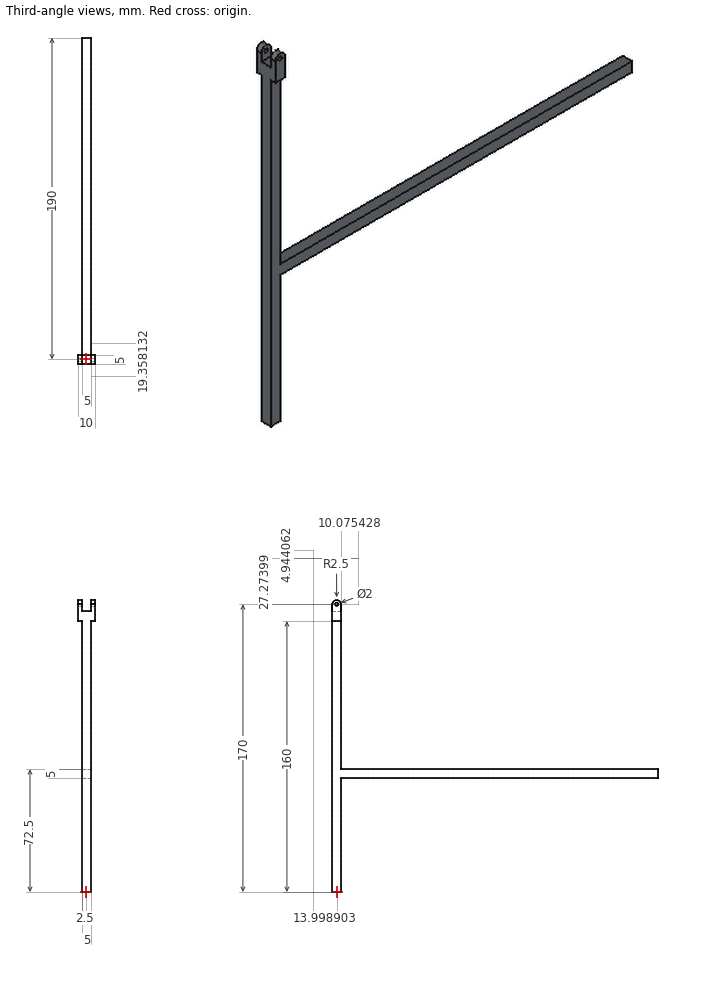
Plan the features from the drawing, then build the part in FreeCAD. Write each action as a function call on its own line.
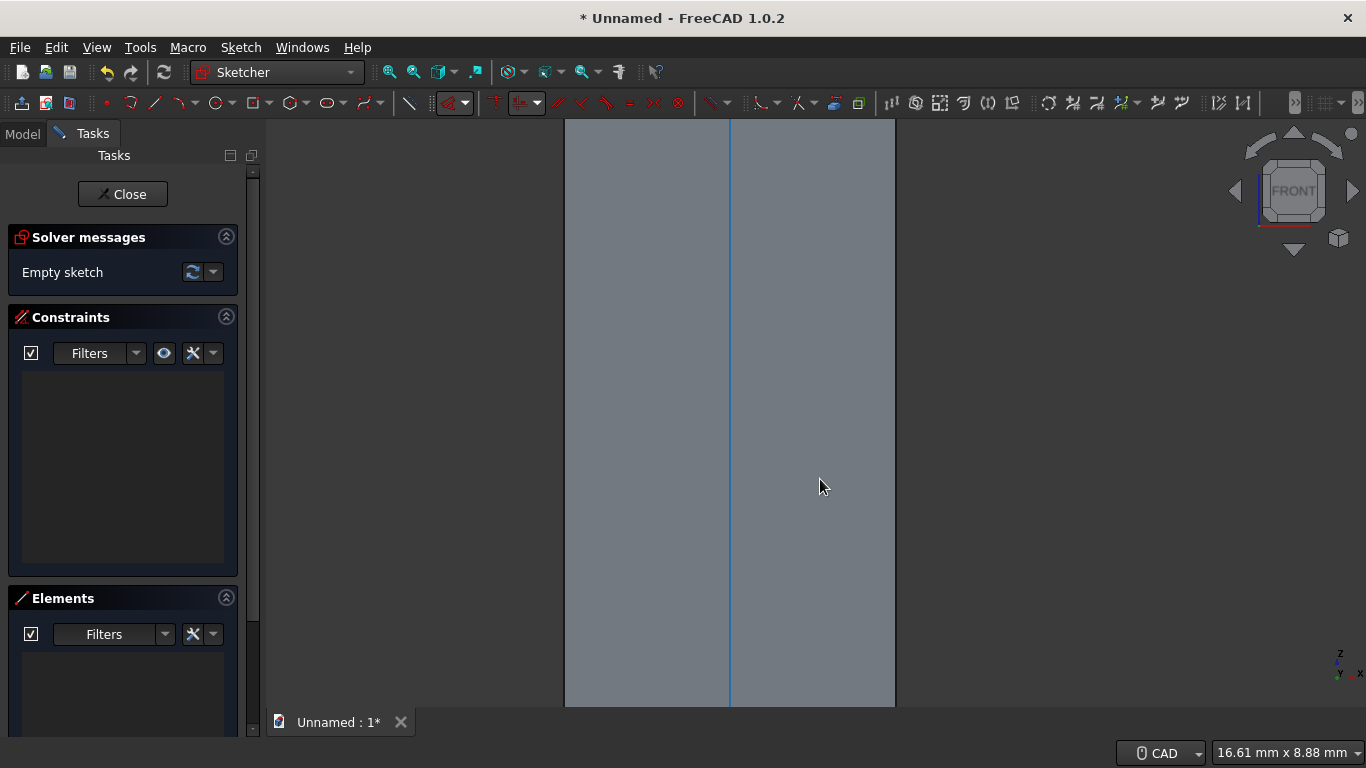
key(g)
key(r)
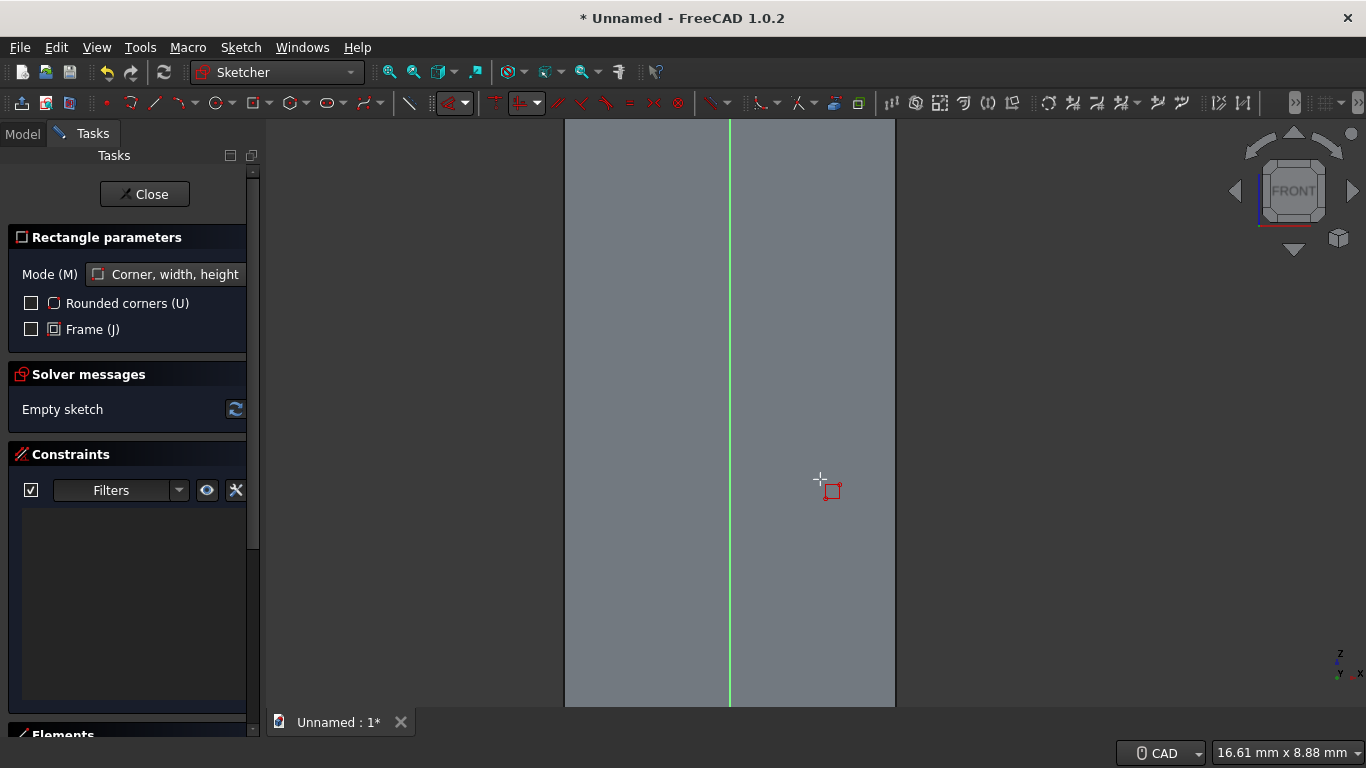
click(564, 234)
click(896, 565)
key(Escape)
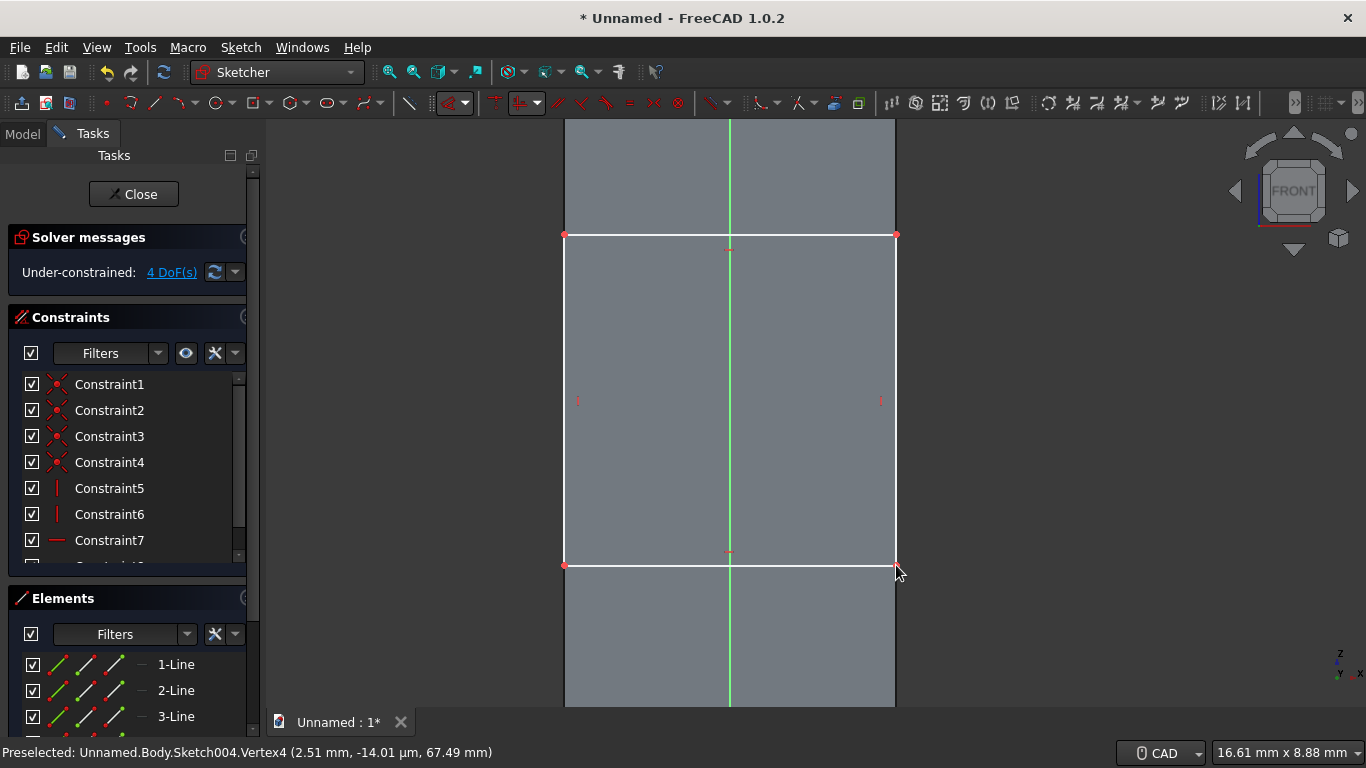
click(564, 334)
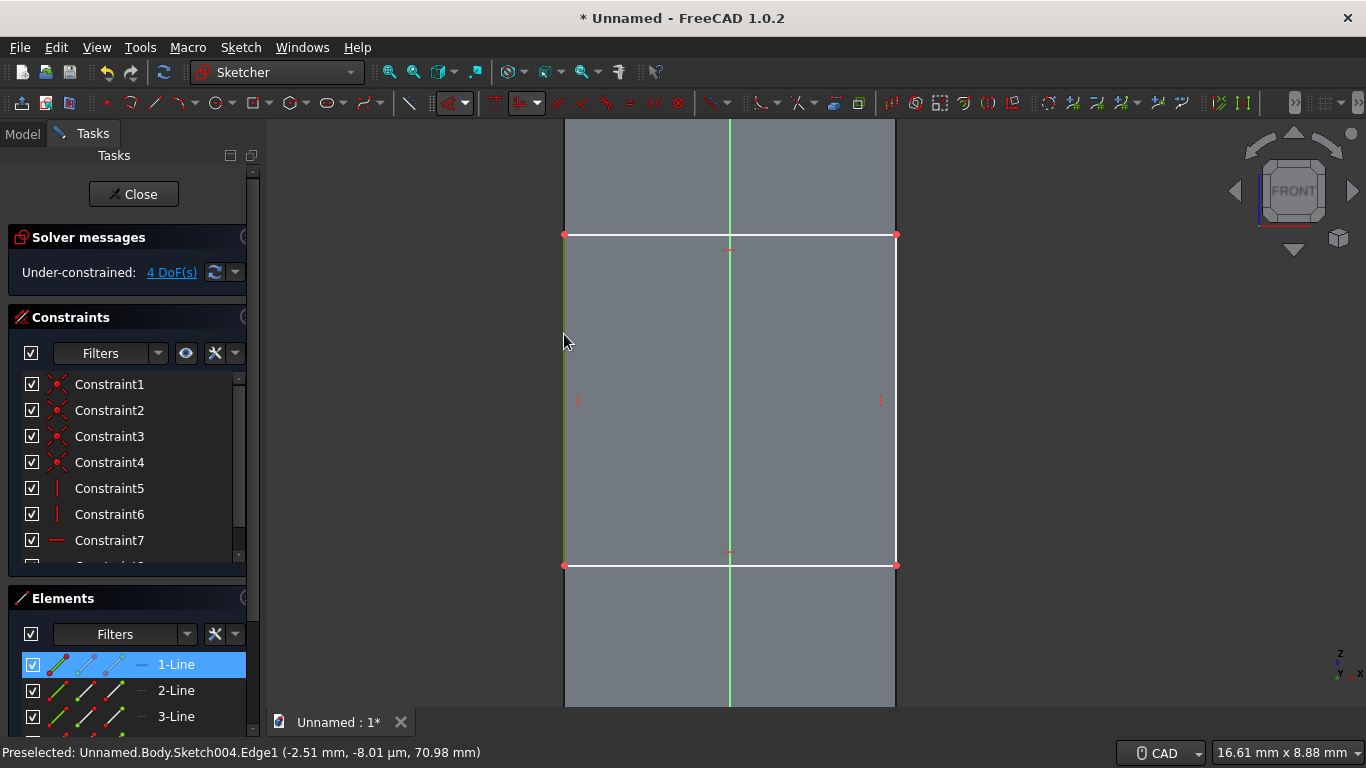
key(i)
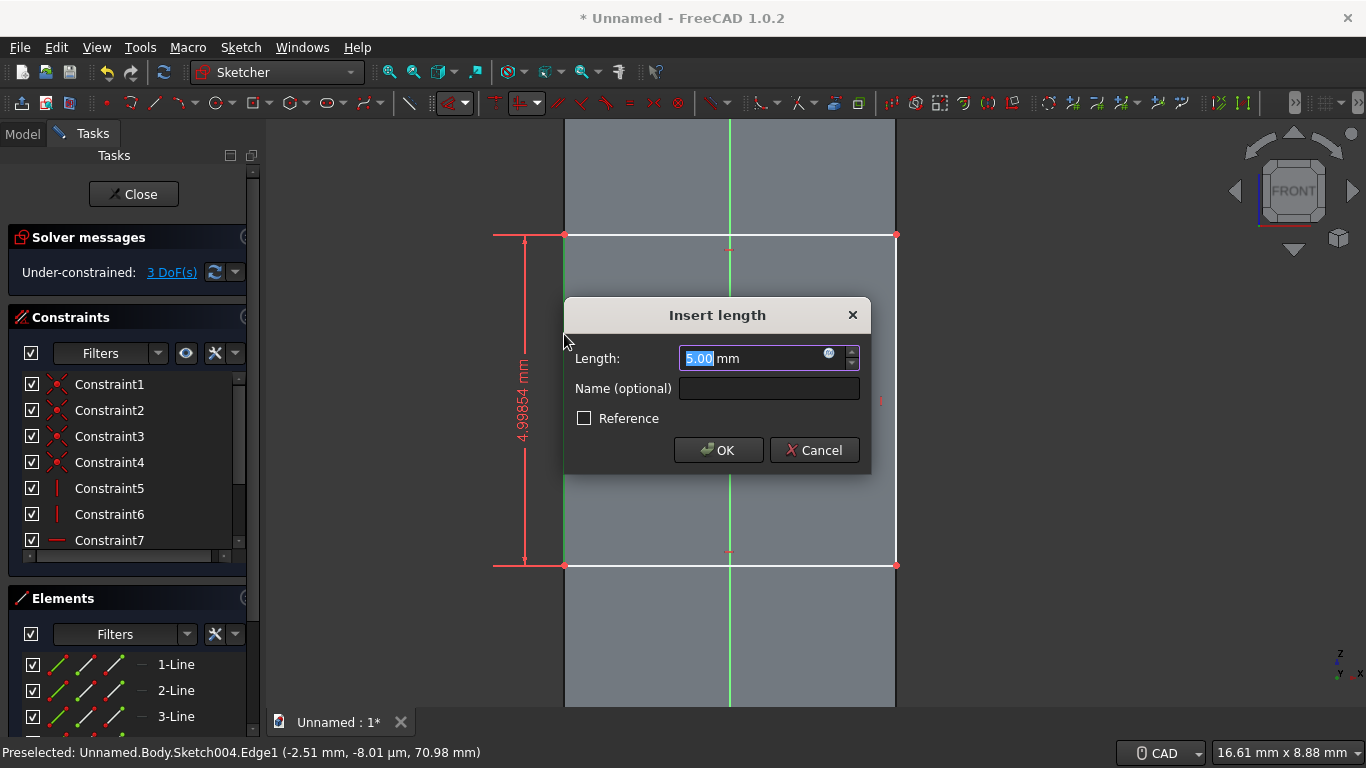
text(5)
key(Return)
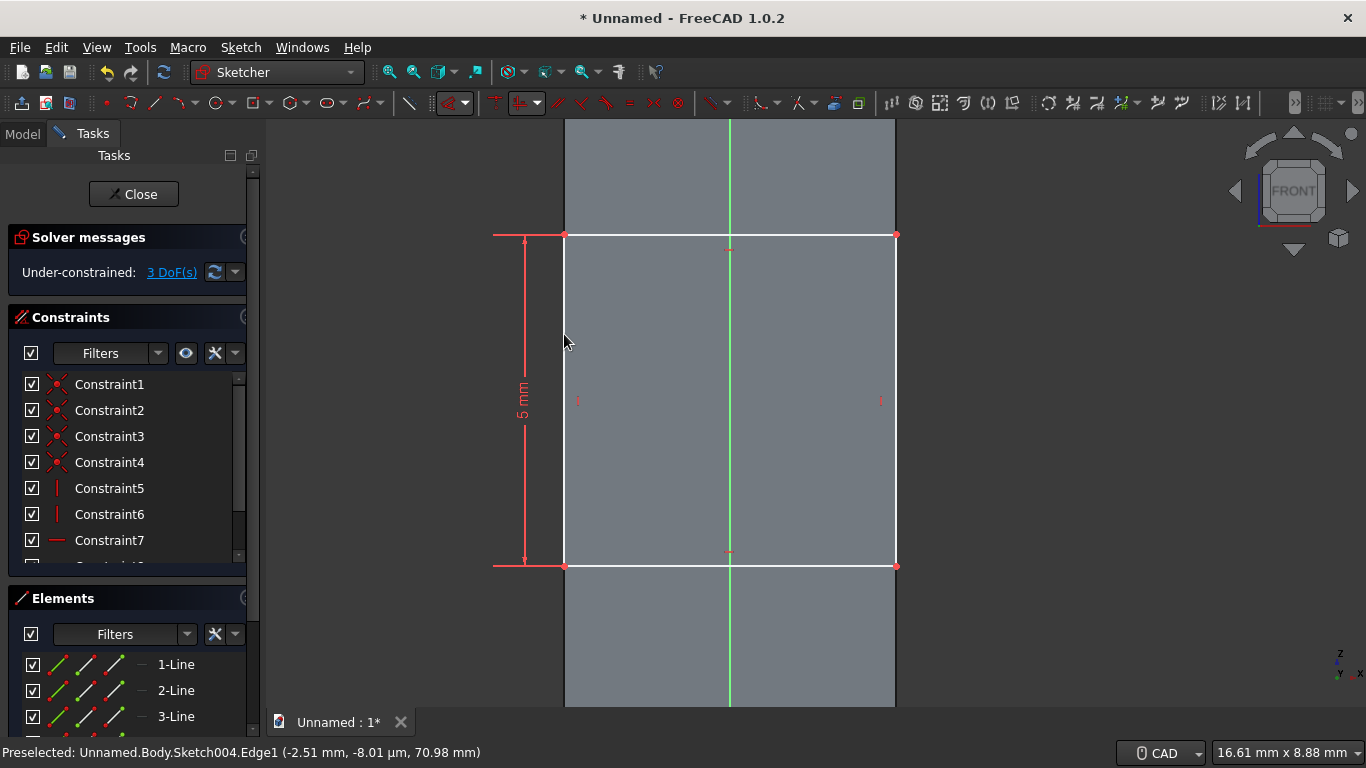
click(664, 566)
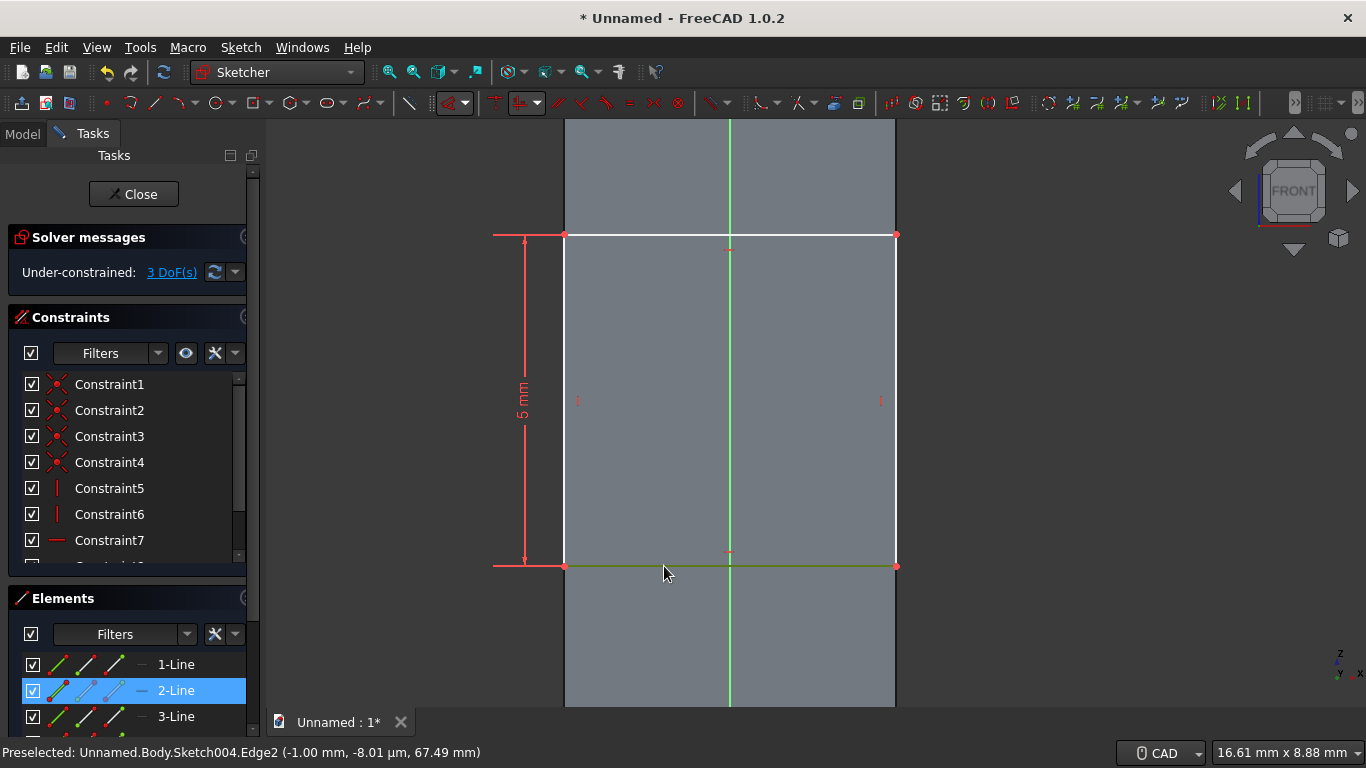
click(468, 104)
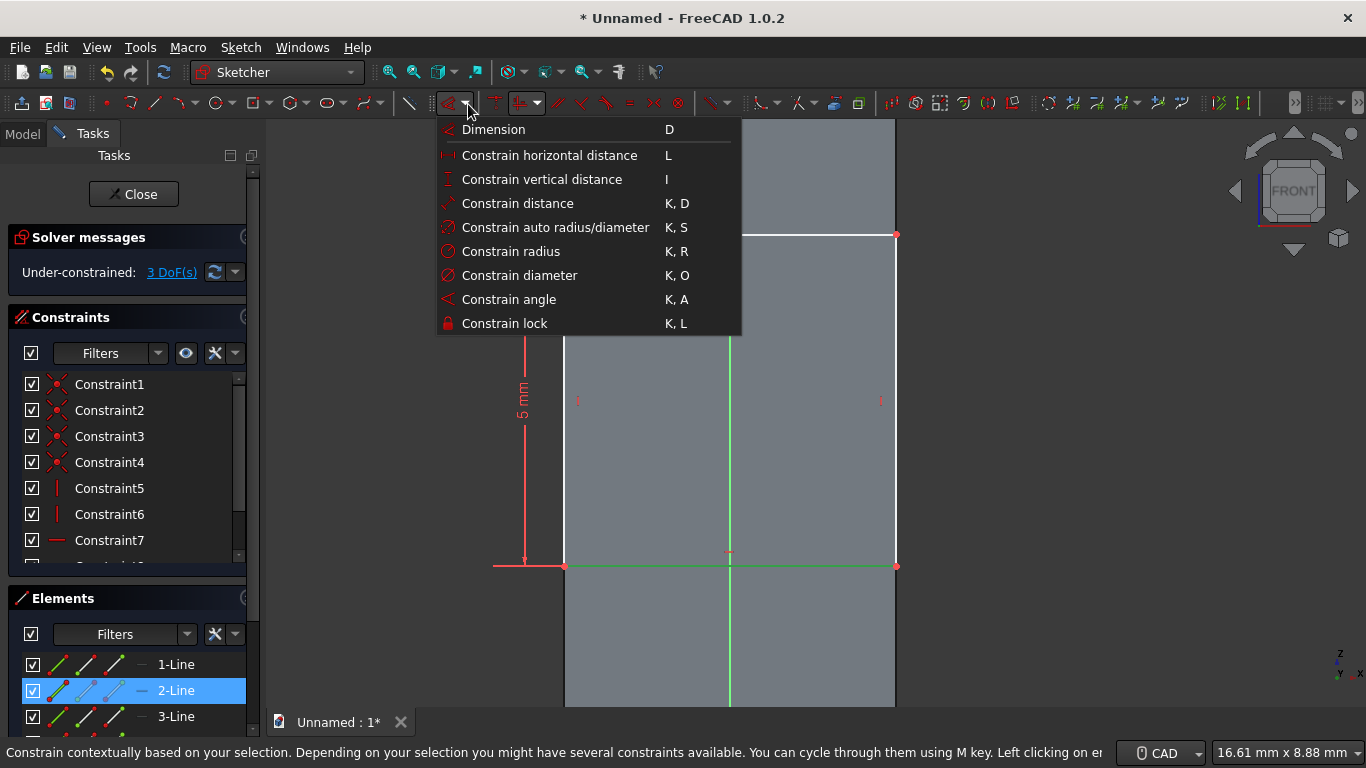
click(589, 155)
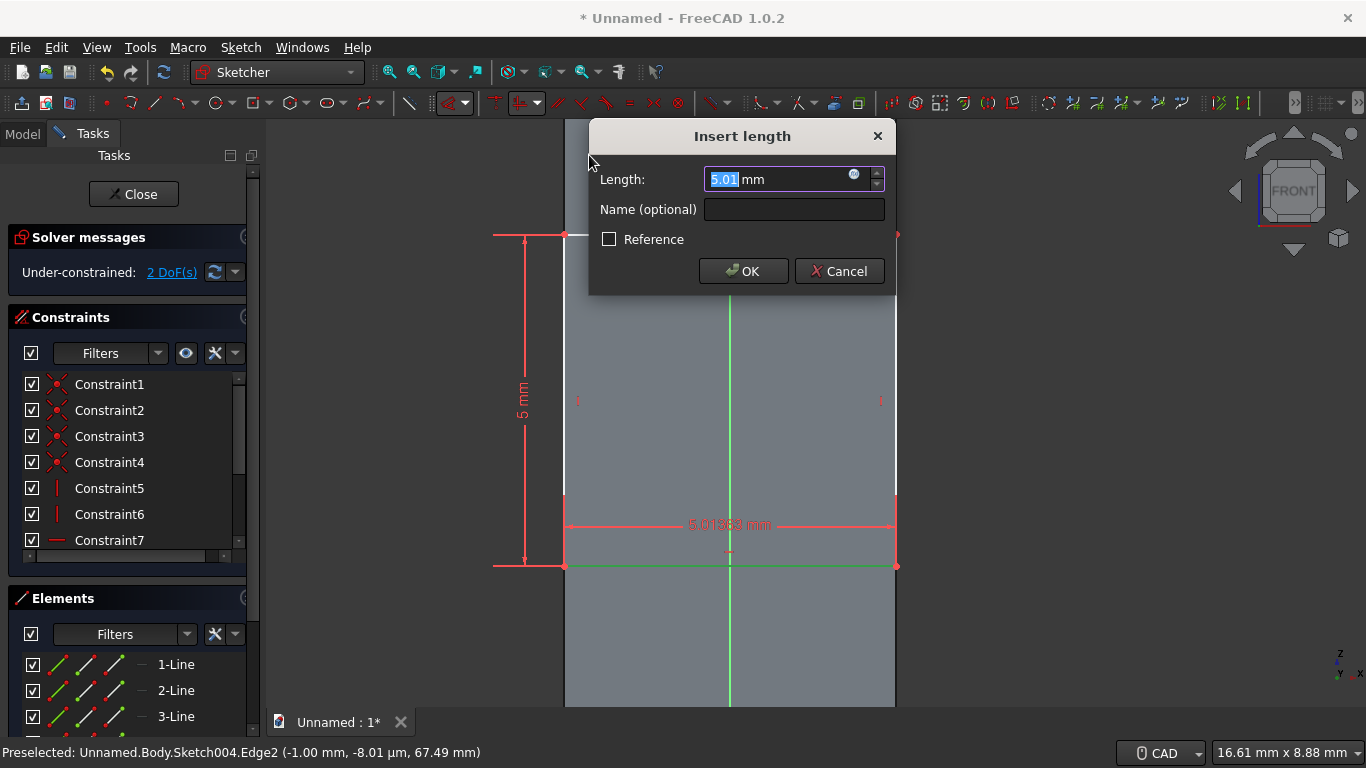
text(5)
key(Return)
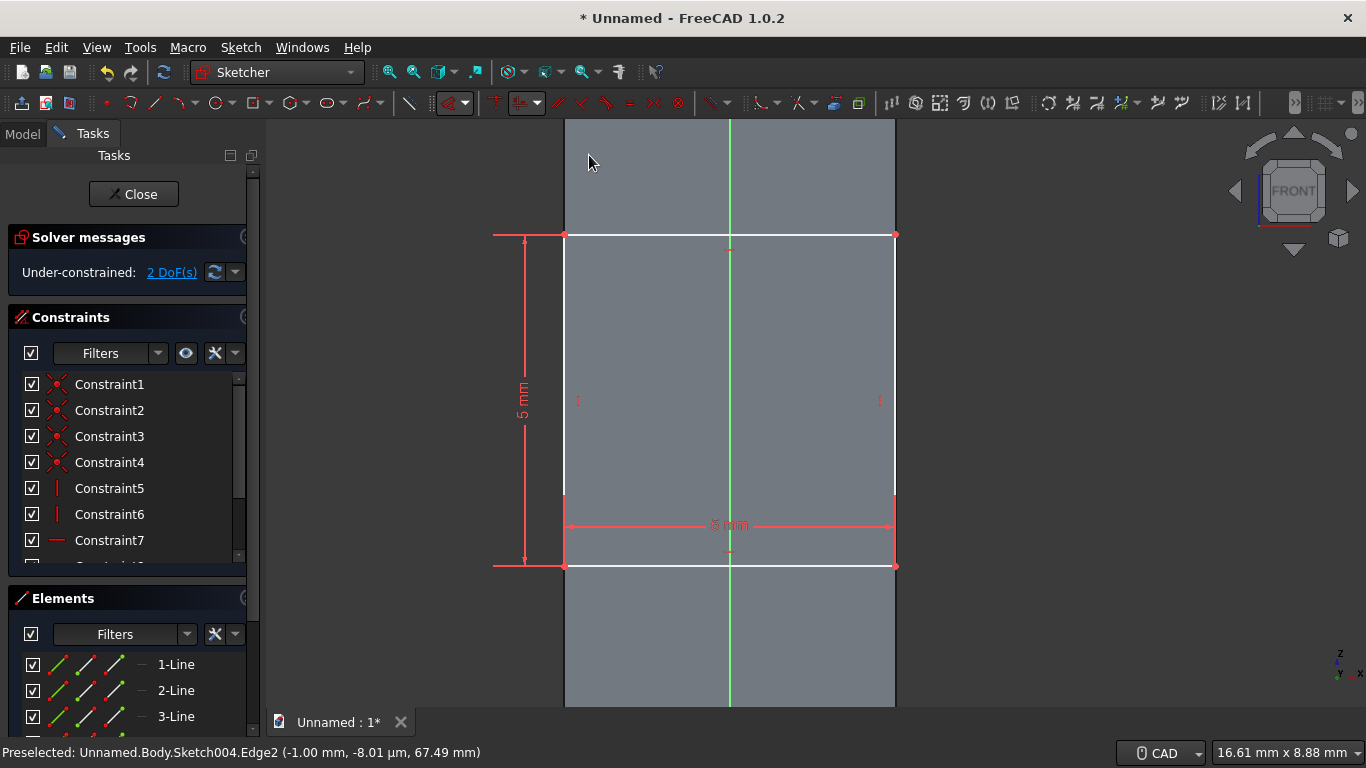
click(564, 235)